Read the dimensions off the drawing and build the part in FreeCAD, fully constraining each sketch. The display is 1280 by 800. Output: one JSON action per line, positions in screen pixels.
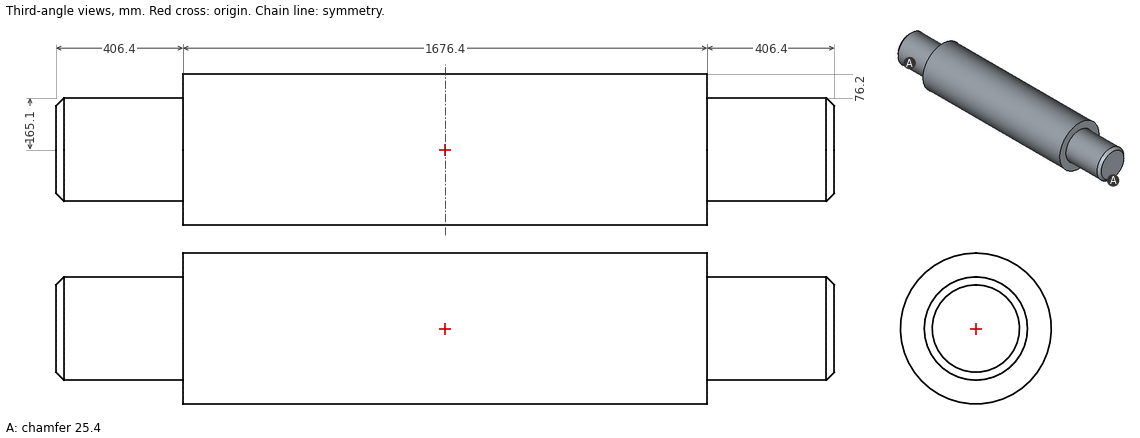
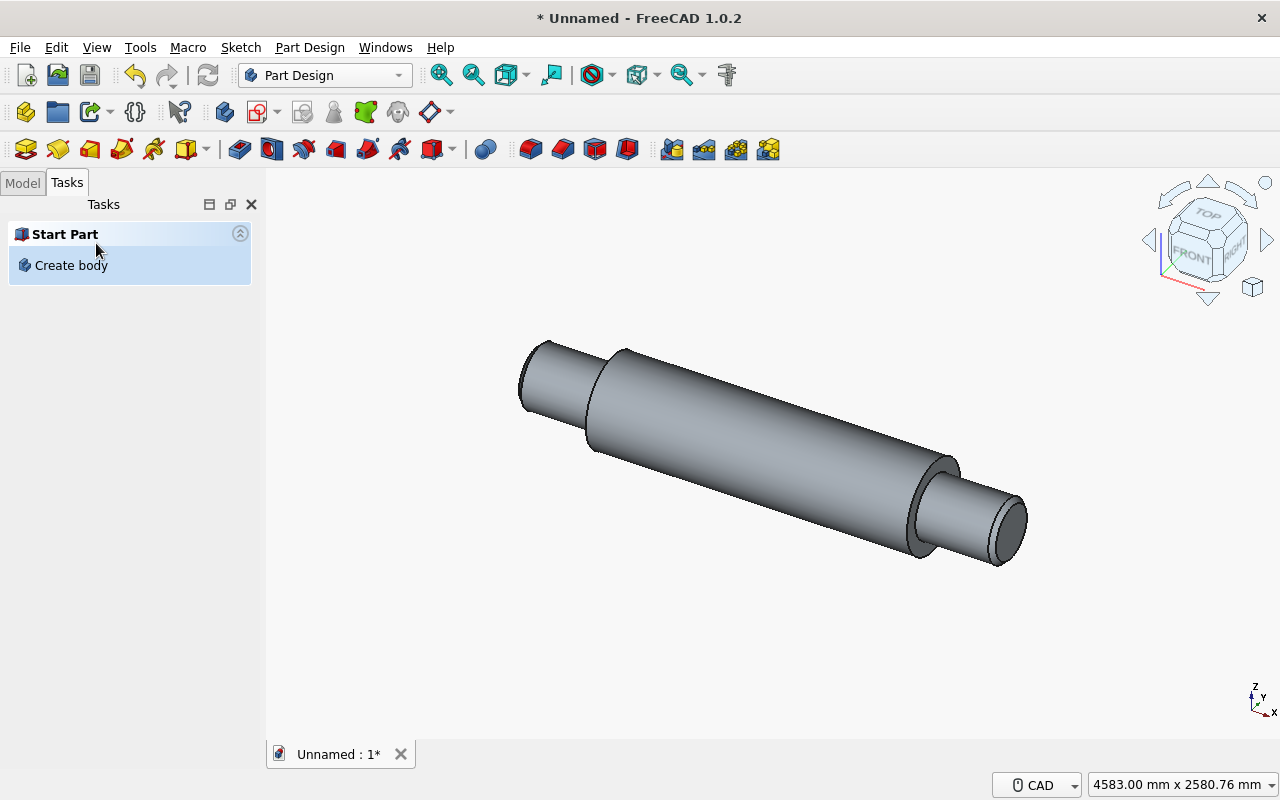
{"action": "key", "text": "0"}